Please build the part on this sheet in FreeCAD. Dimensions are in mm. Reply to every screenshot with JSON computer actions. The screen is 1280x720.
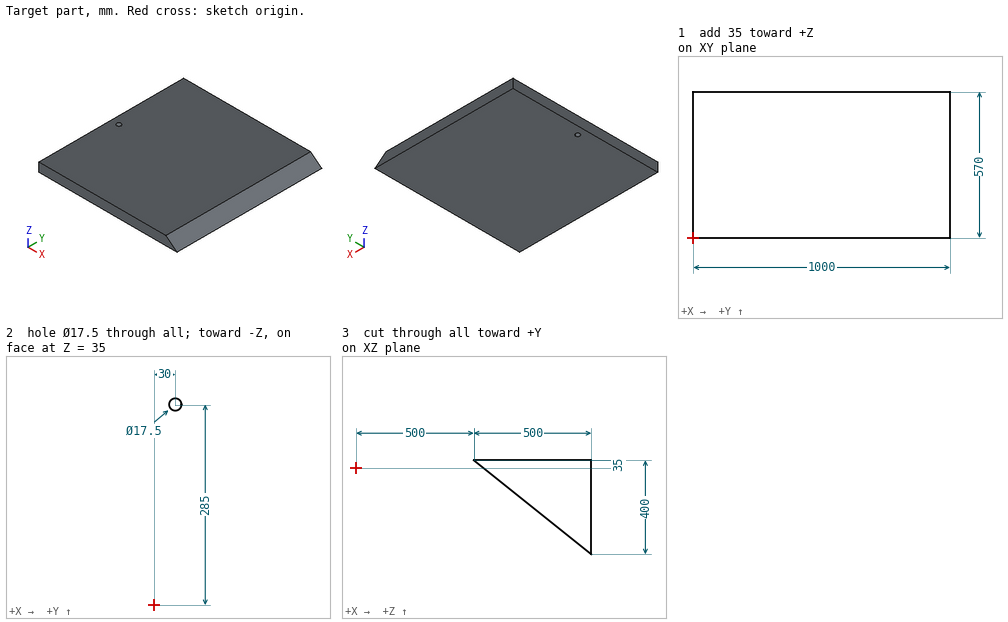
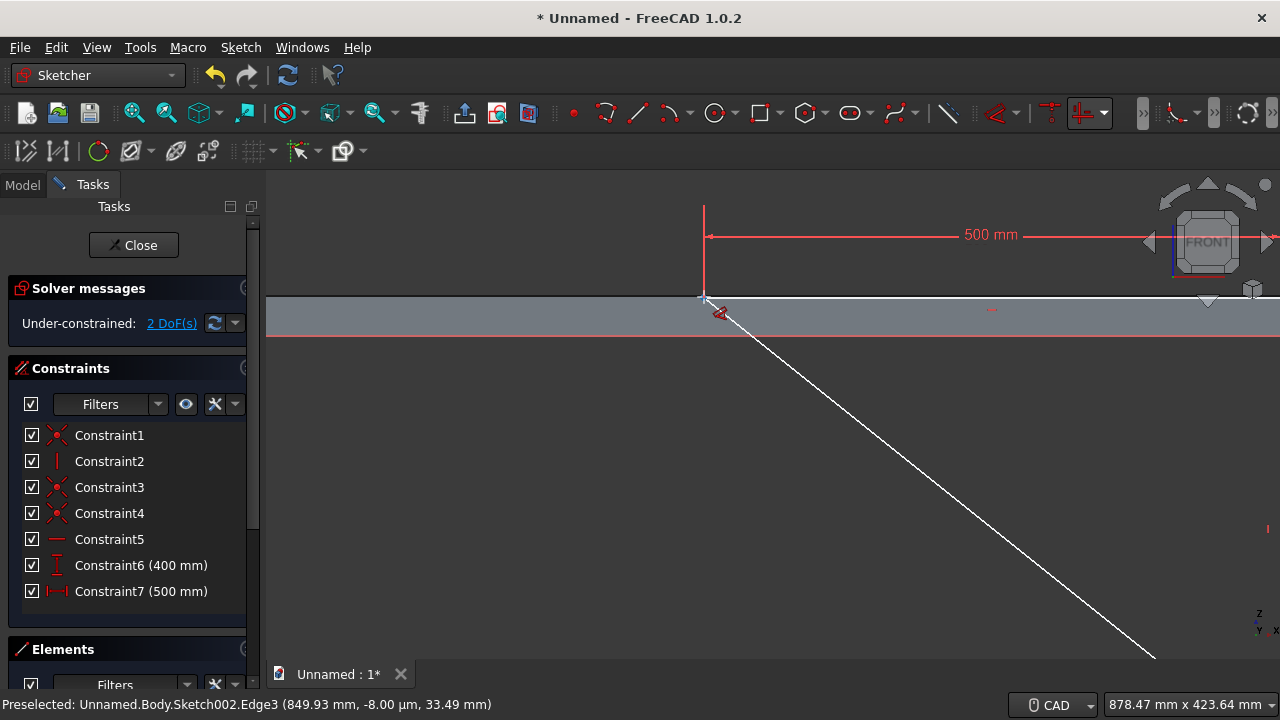
{"action": "left_click", "coordinate": [704, 298]}
{"action": "left_click", "coordinate": [762, 317]}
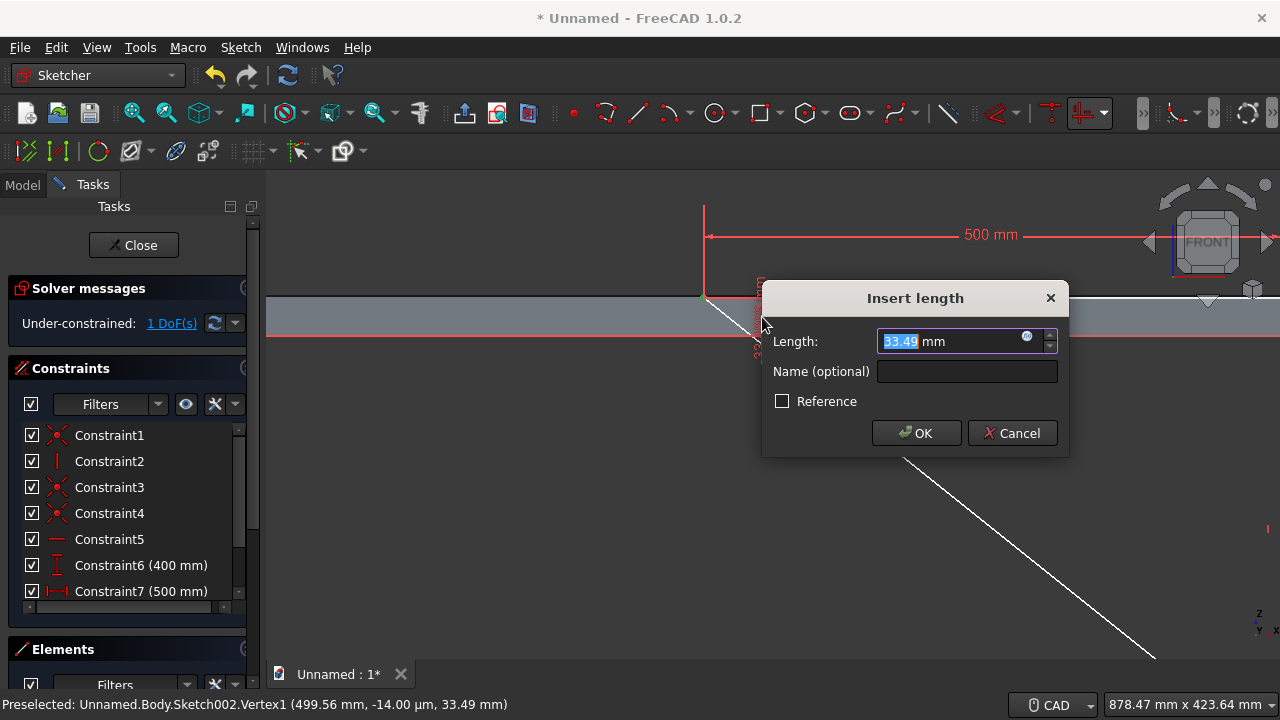
{"action": "type", "text": "35"}
{"action": "key", "text": "Return"}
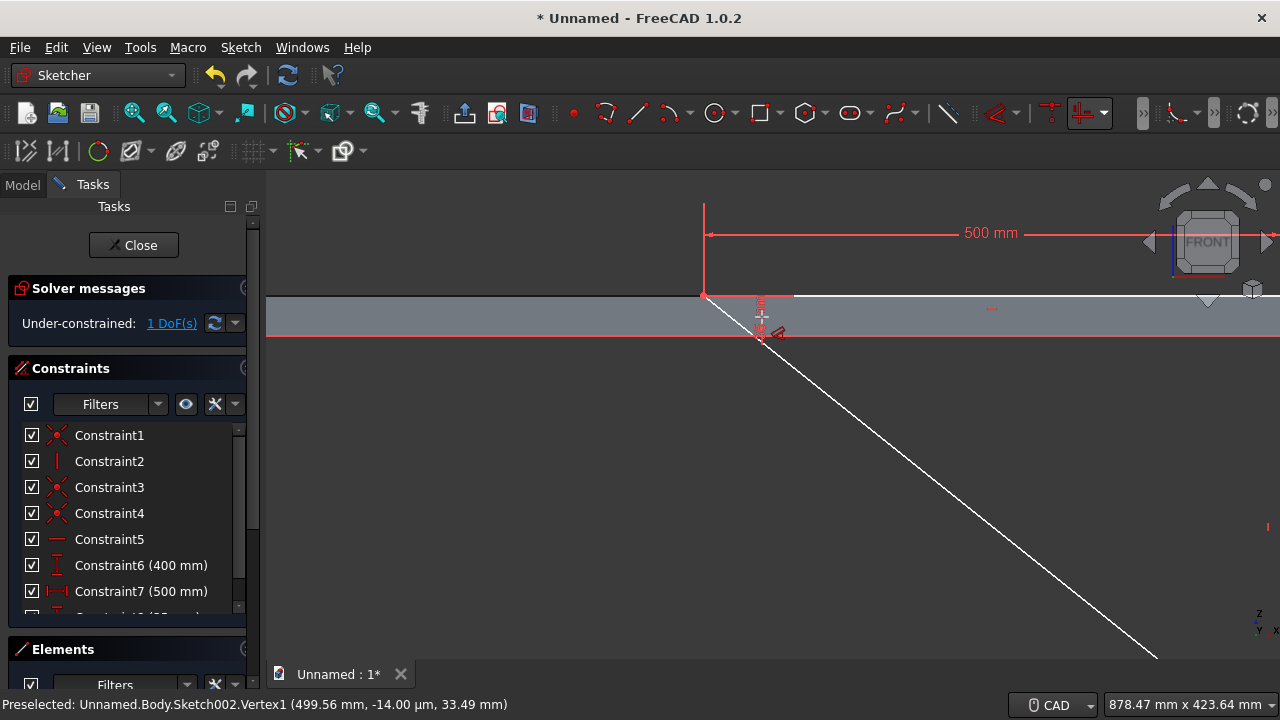
{"action": "left_click", "coordinate": [704, 296]}
{"action": "left_click", "coordinate": [499, 262]}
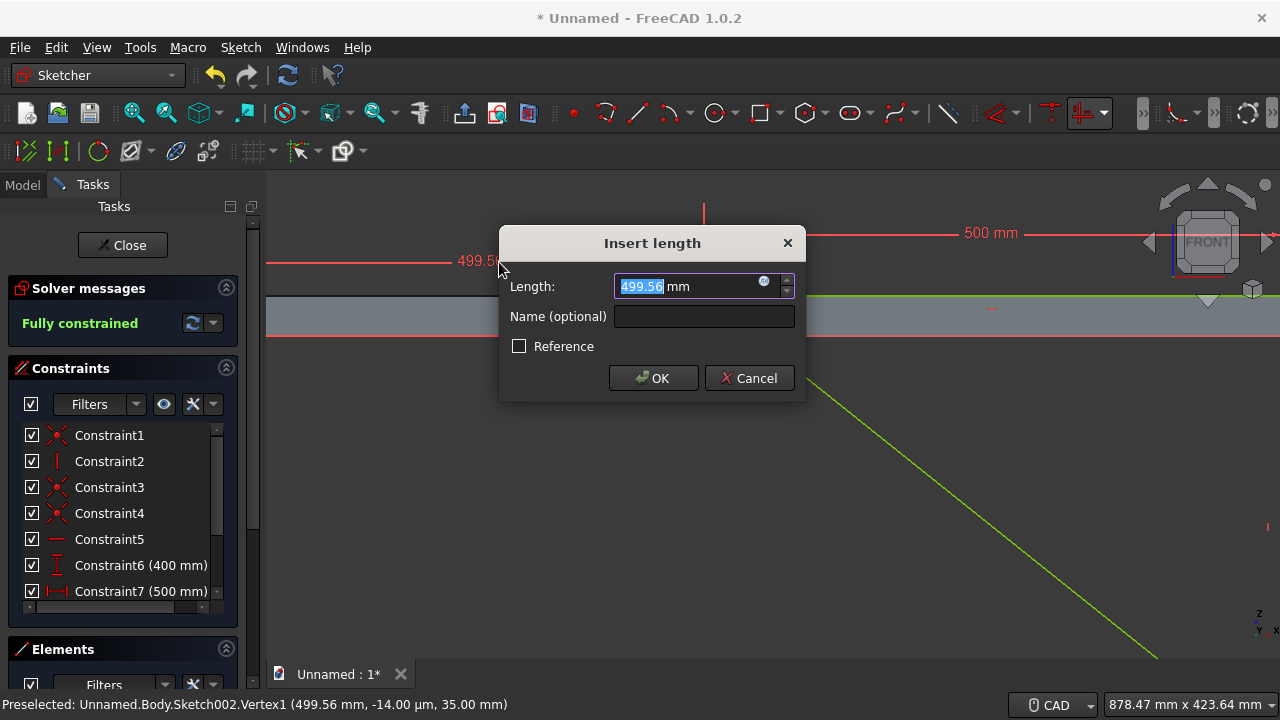
{"action": "type", "text": "500"}
{"action": "key", "text": "Return"}
{"action": "key", "text": "Escape"}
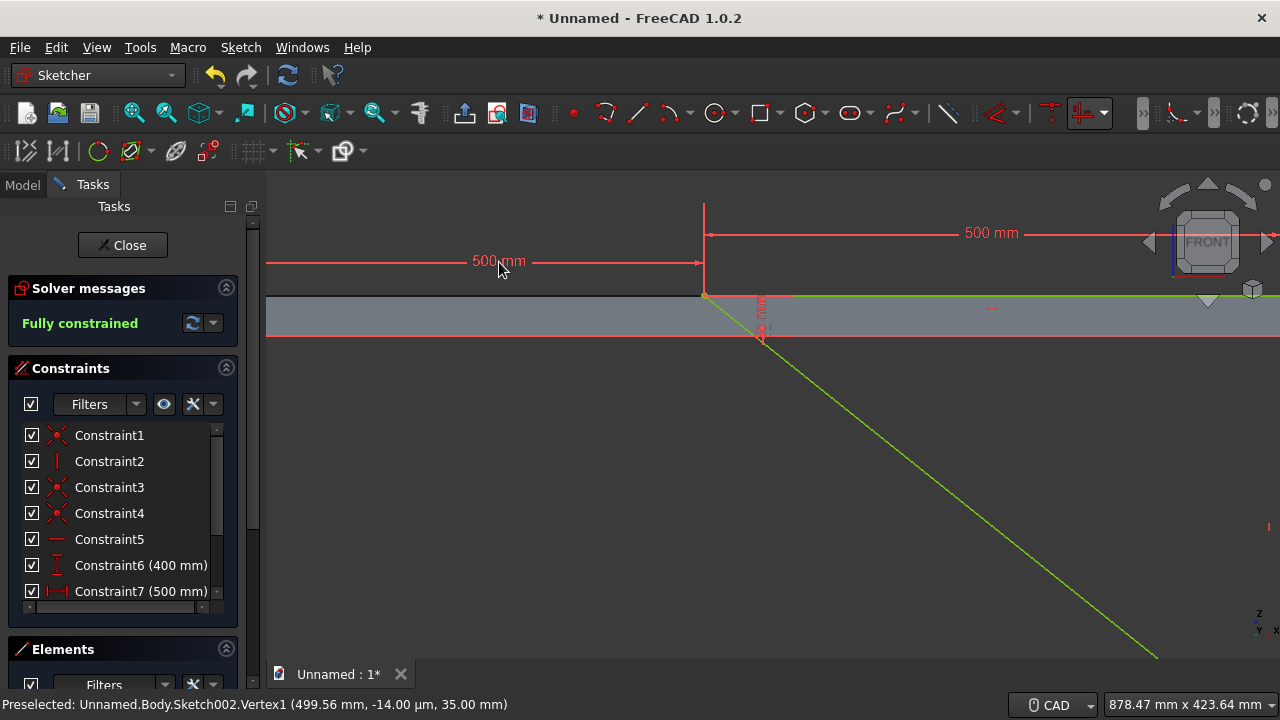
{"action": "left_click", "coordinate": [123, 245]}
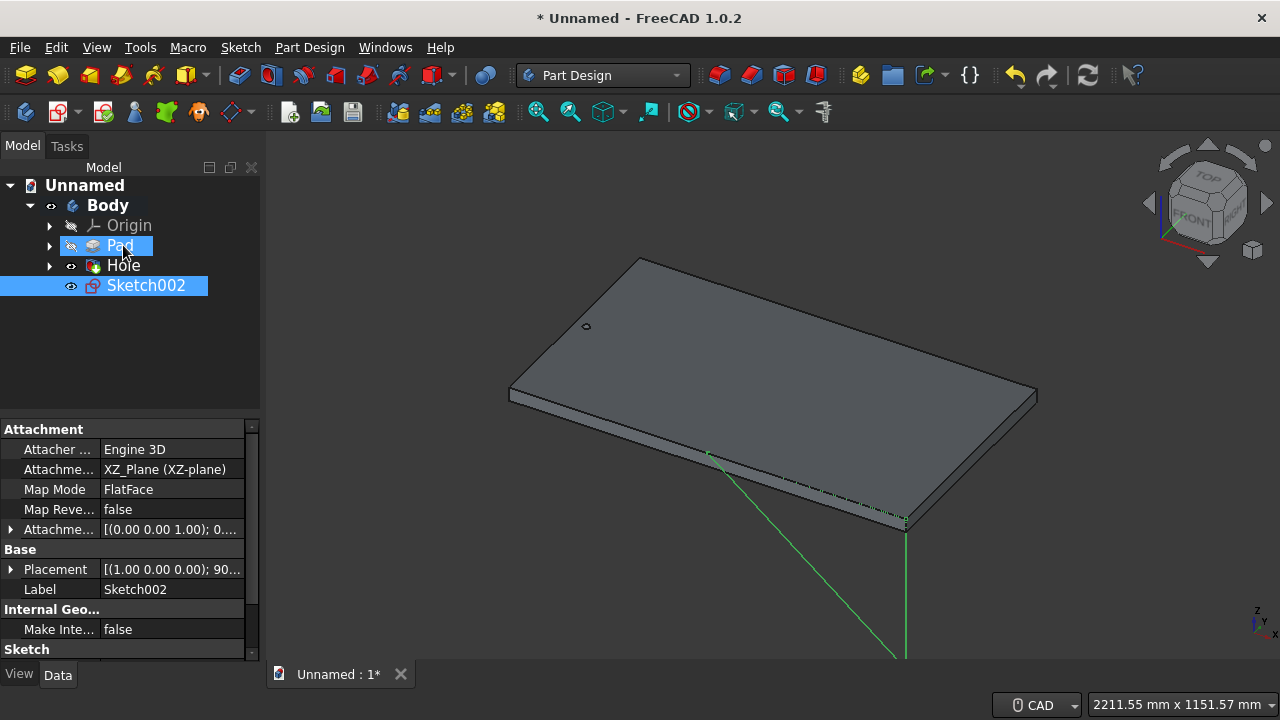
{"action": "left_click", "coordinate": [240, 76]}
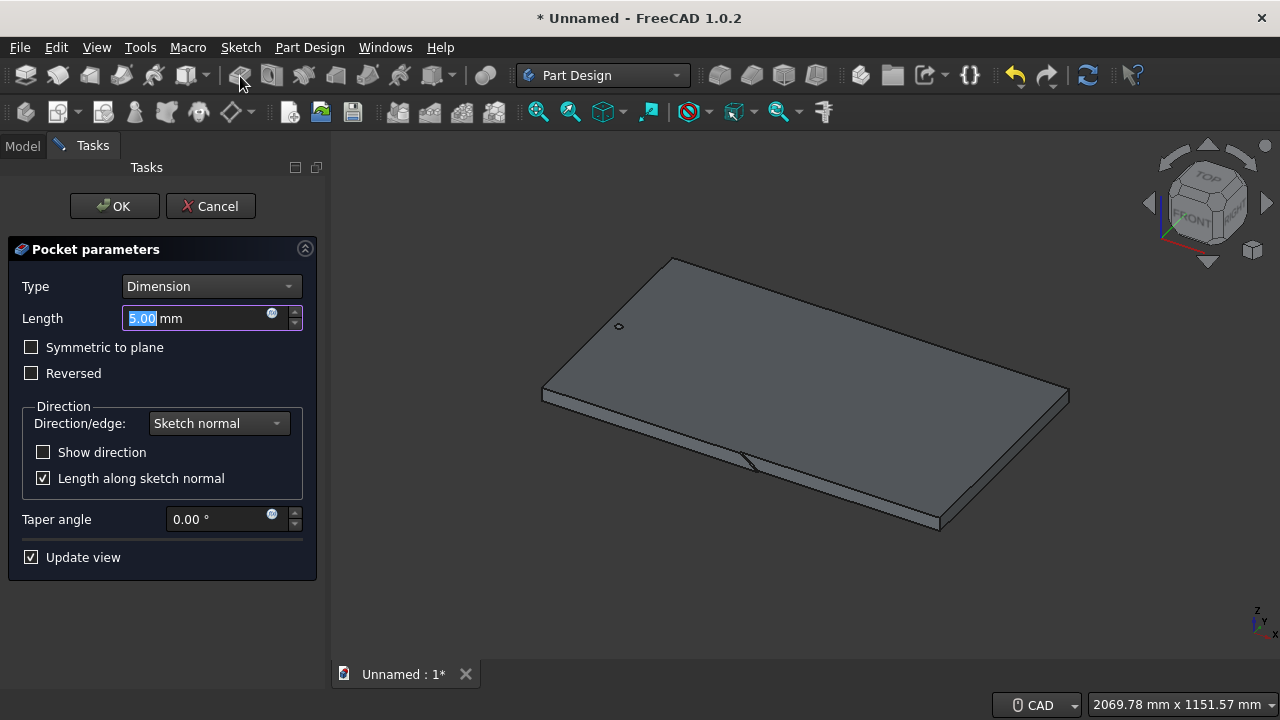
{"action": "left_click", "coordinate": [212, 286]}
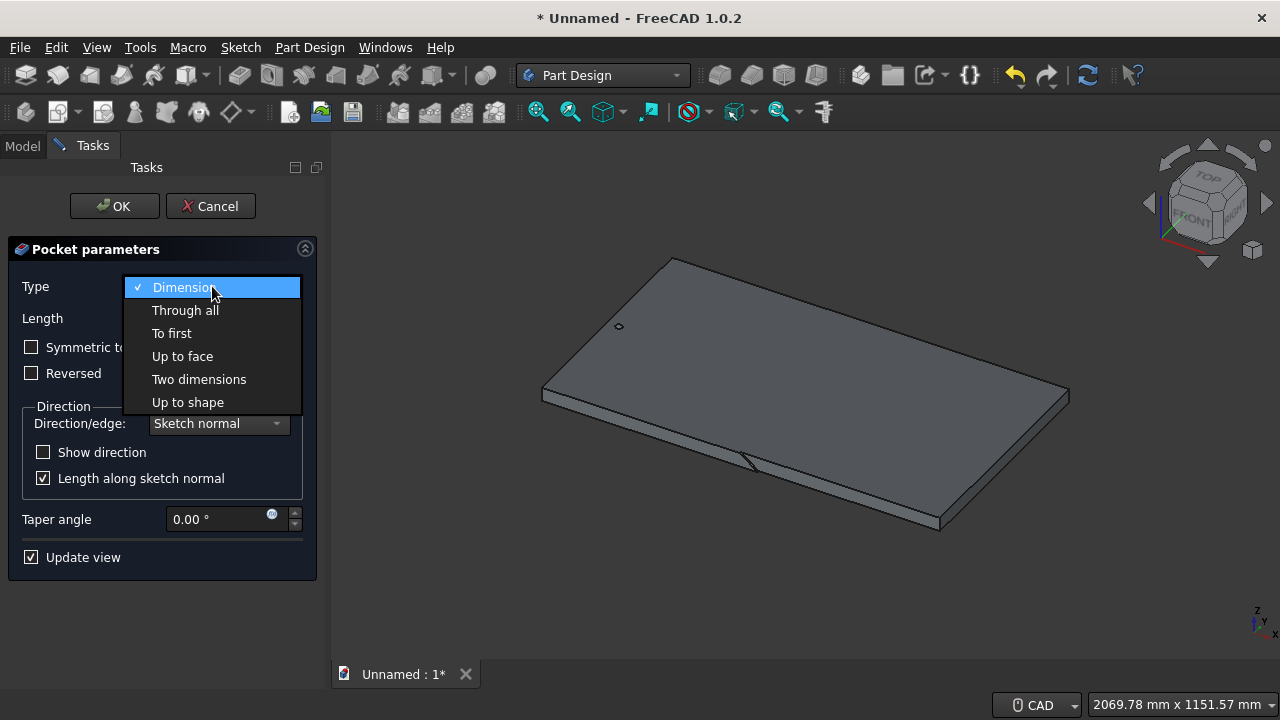
{"action": "left_click", "coordinate": [212, 310]}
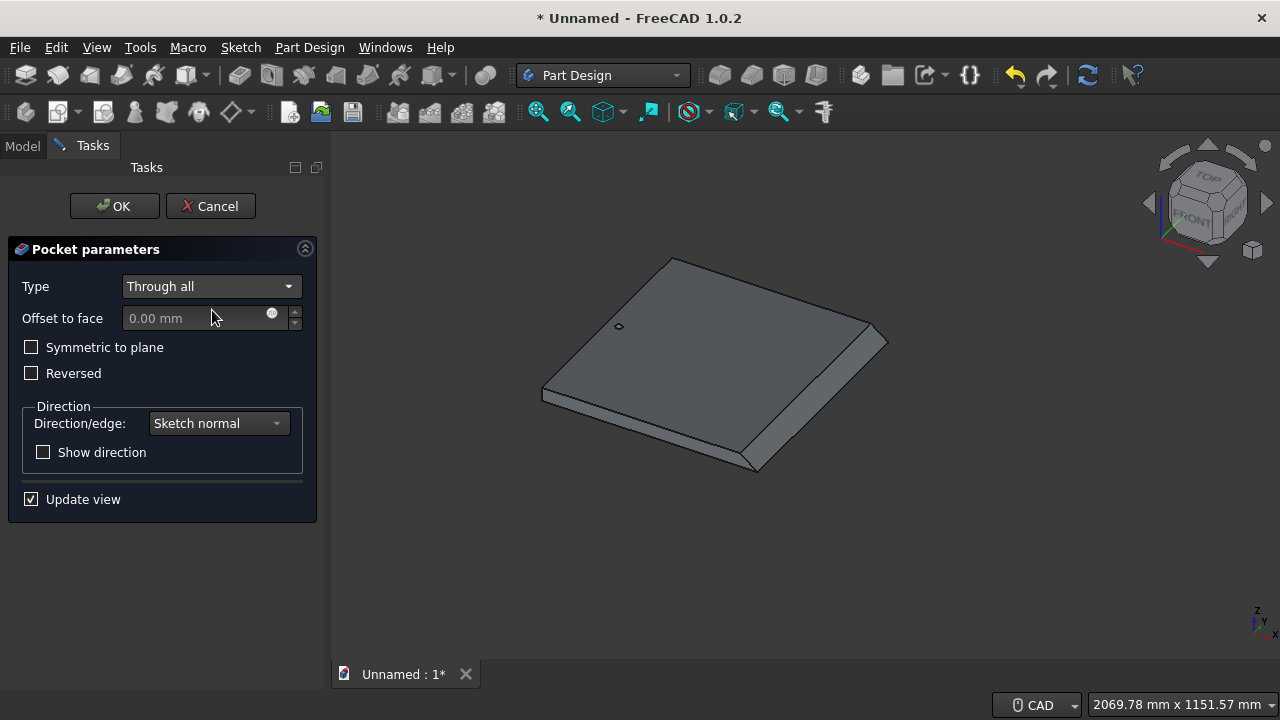
{"action": "left_click", "coordinate": [115, 206]}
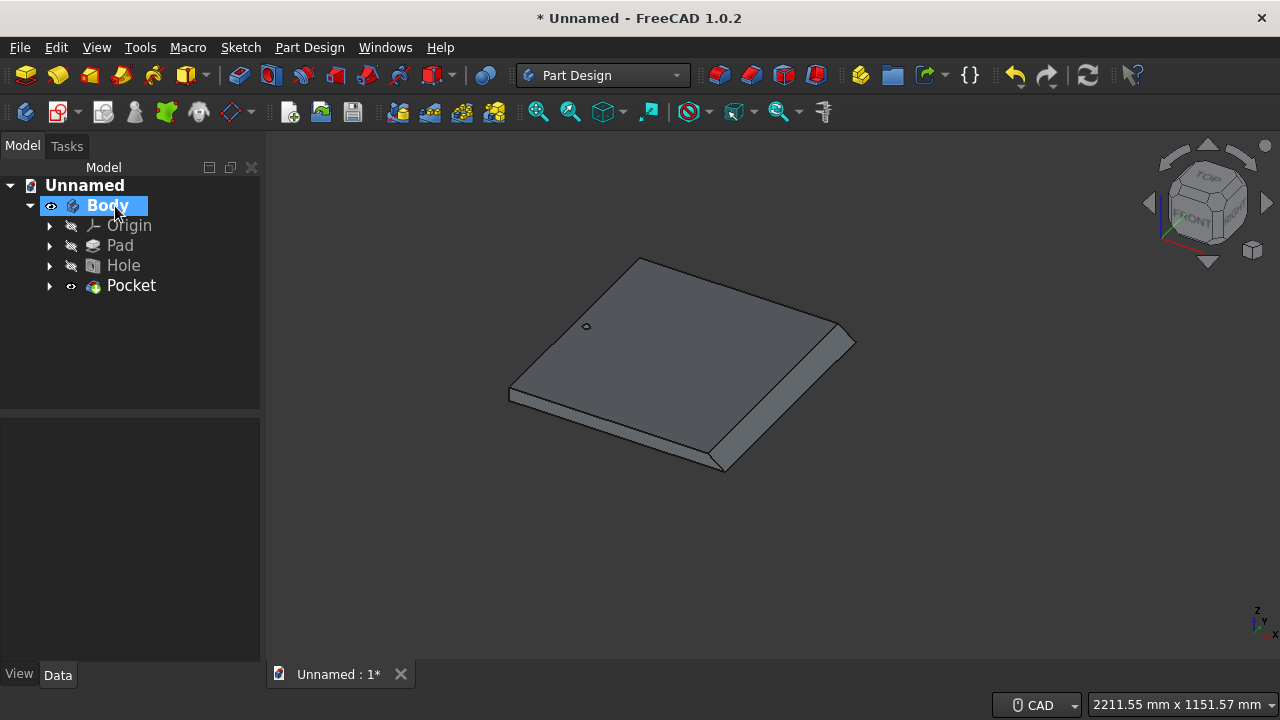
{"action": "key", "text": "0"}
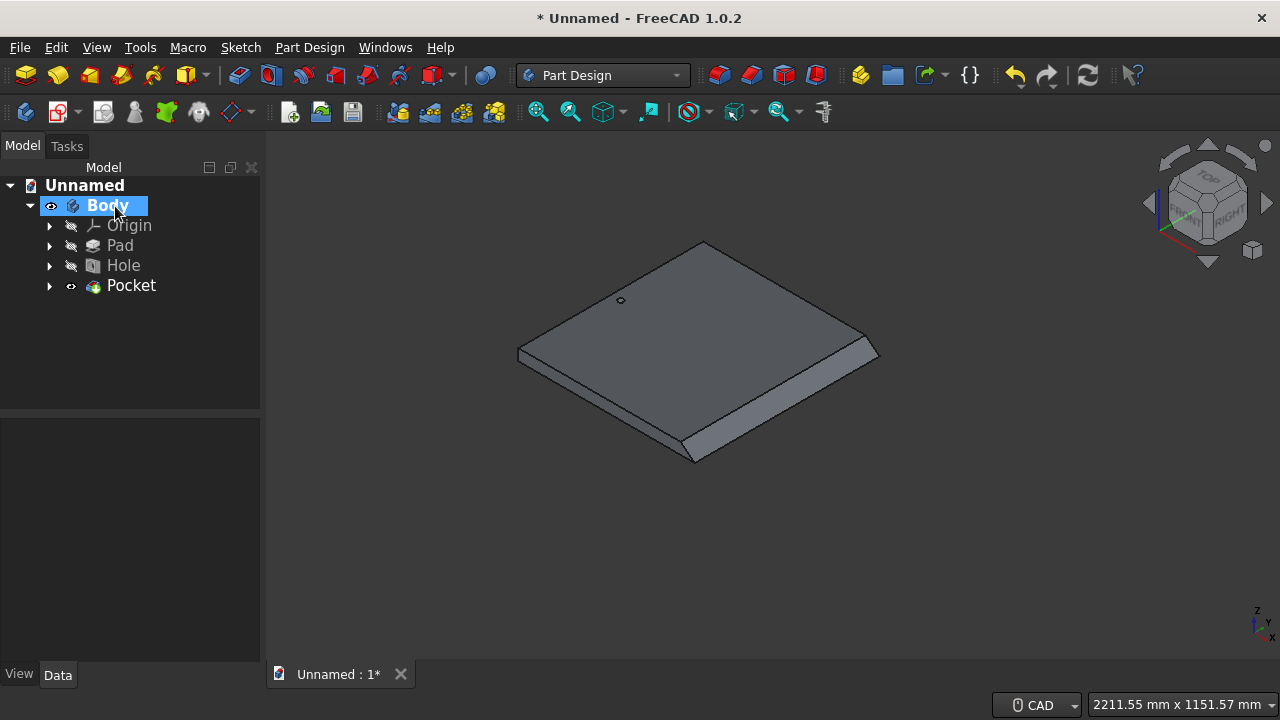
{"action": "left_click", "coordinate": [540, 112]}